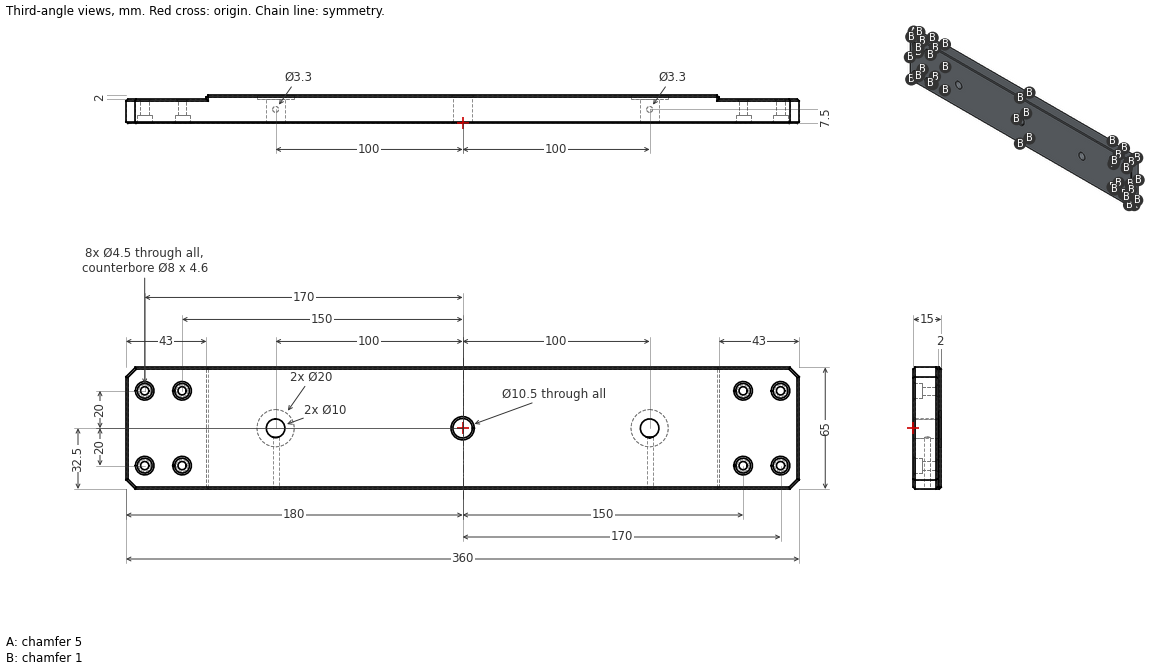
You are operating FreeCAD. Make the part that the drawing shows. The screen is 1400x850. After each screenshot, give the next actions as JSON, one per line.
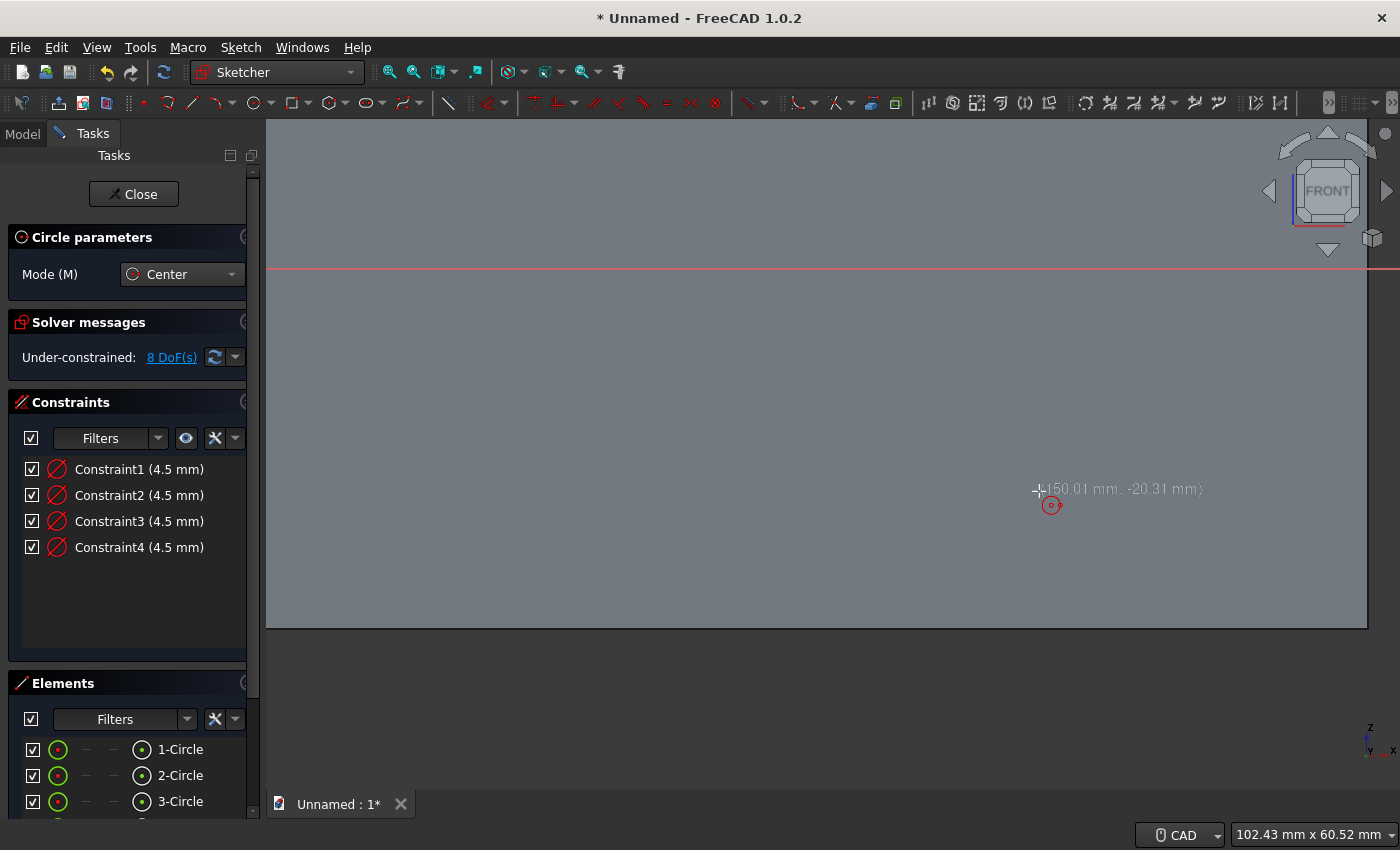
{"action": "scroll", "coordinate": [1040, 491], "scroll_direction": "down", "scroll_amount": 9}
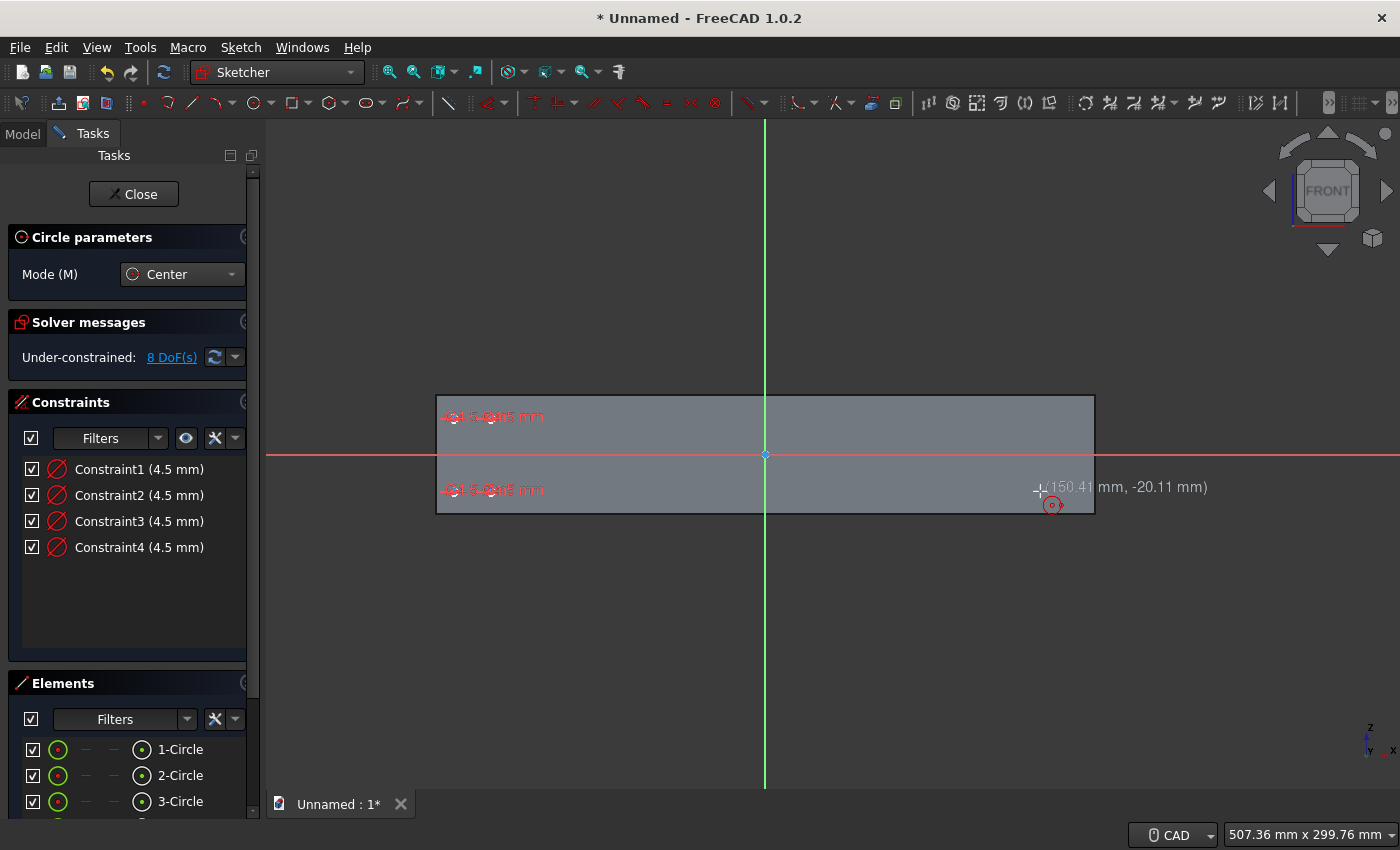
{"action": "left_click", "coordinate": [1040, 491]}
{"action": "mouse_move", "coordinate": [1043, 489]}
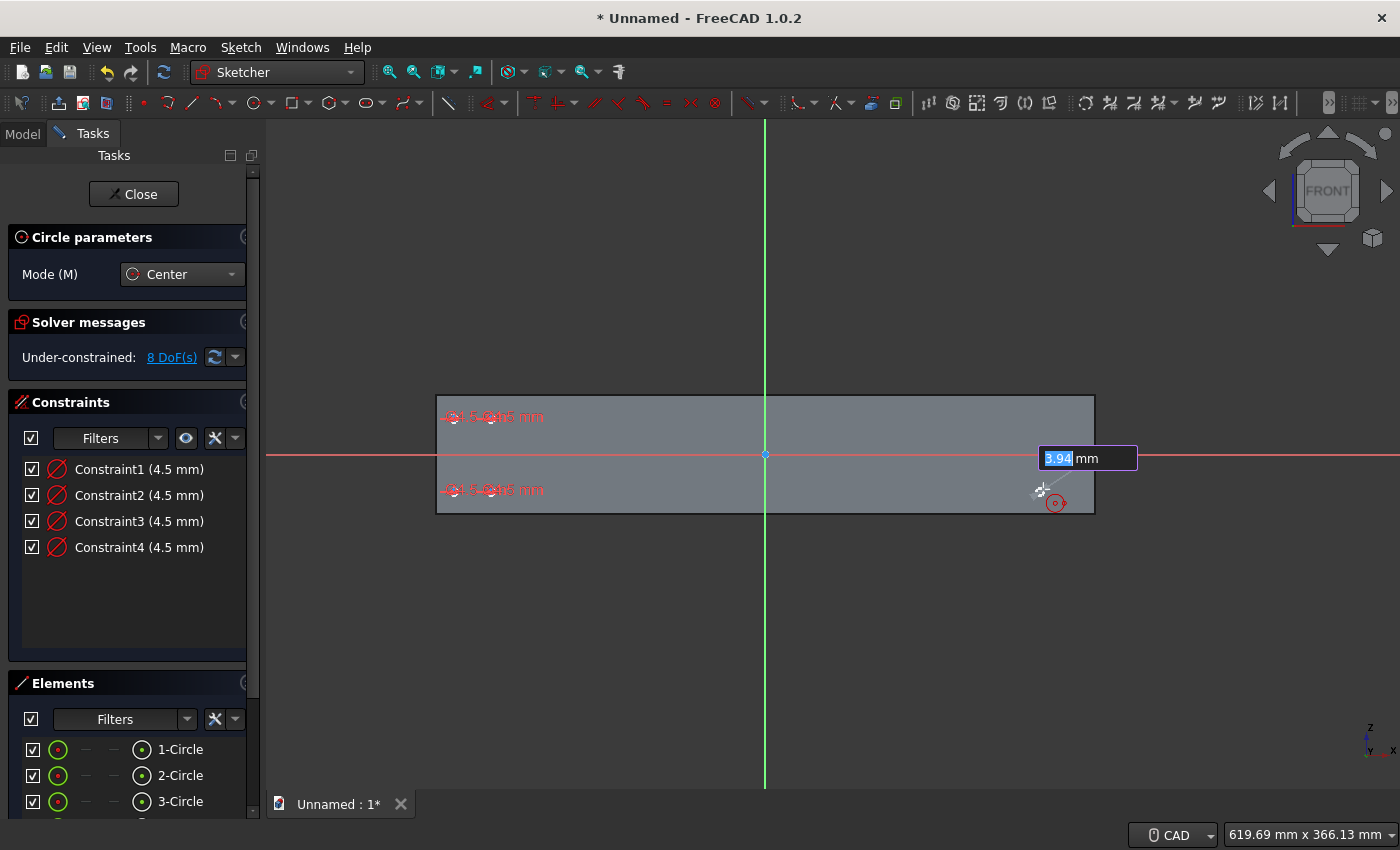
{"action": "type", "text": "4.5"}
{"action": "key", "text": "Return"}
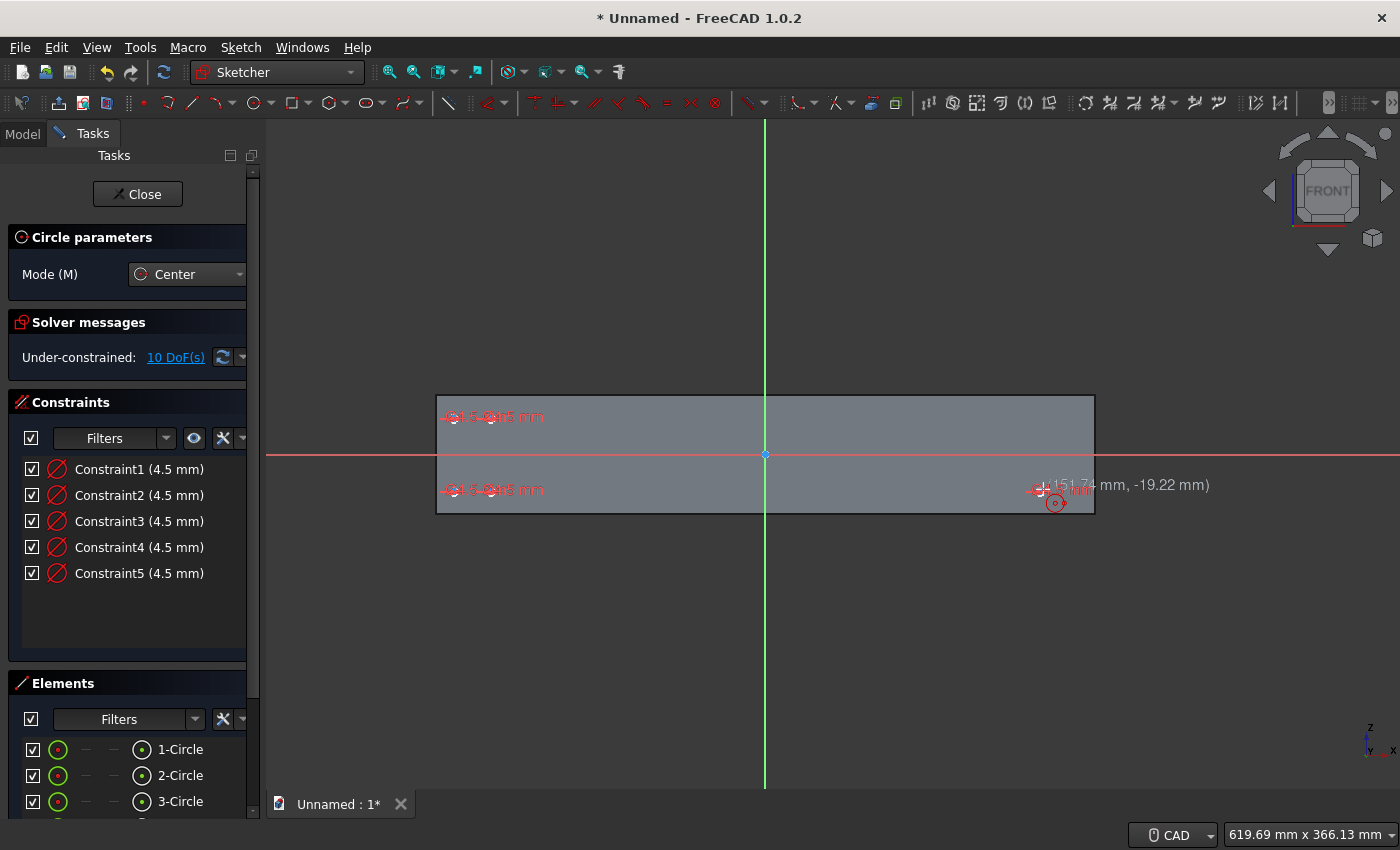
{"action": "scroll", "coordinate": [1076, 491], "scroll_direction": "up", "scroll_amount": 9}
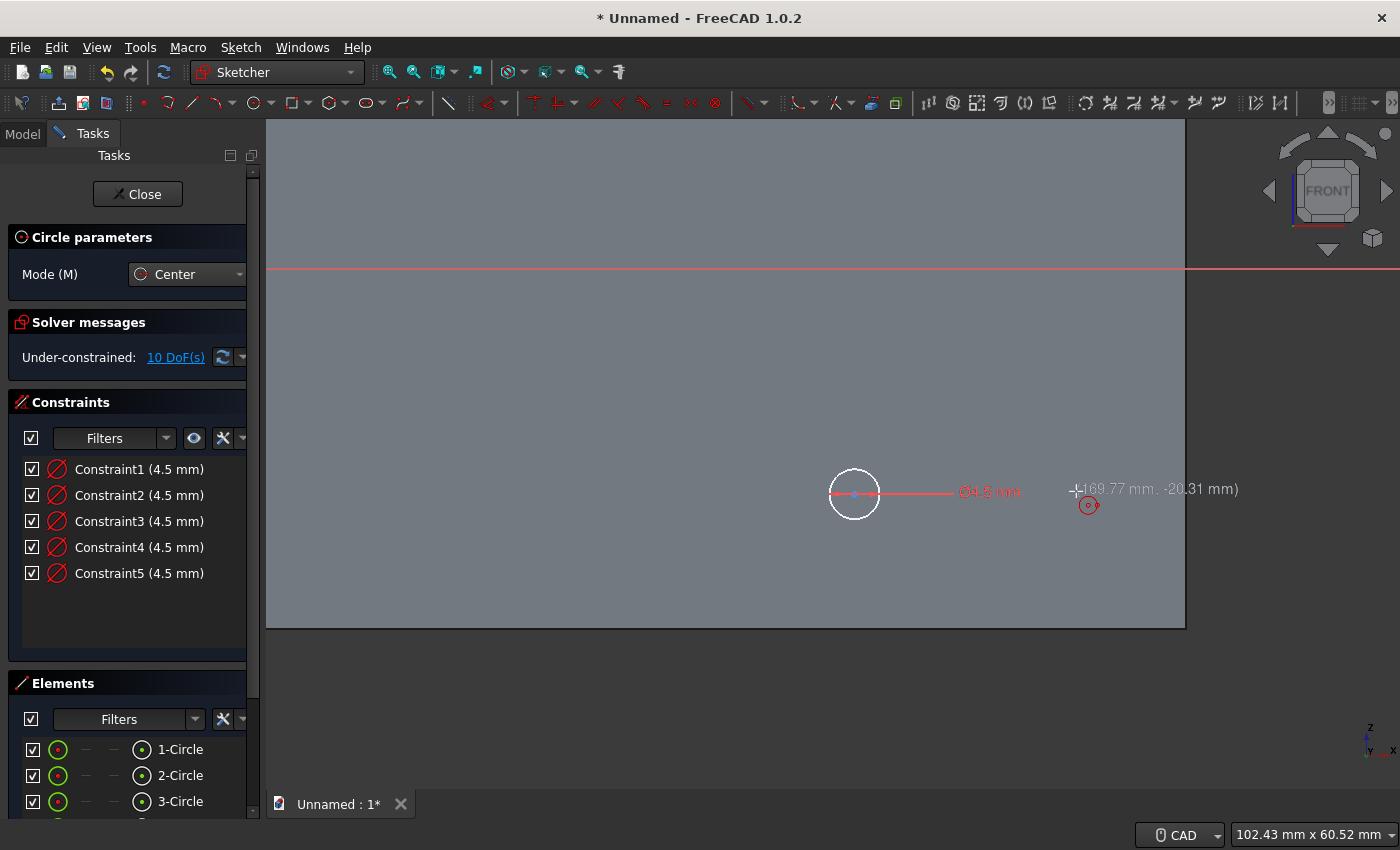
{"action": "scroll", "coordinate": [1076, 491], "scroll_direction": "down", "scroll_amount": 9}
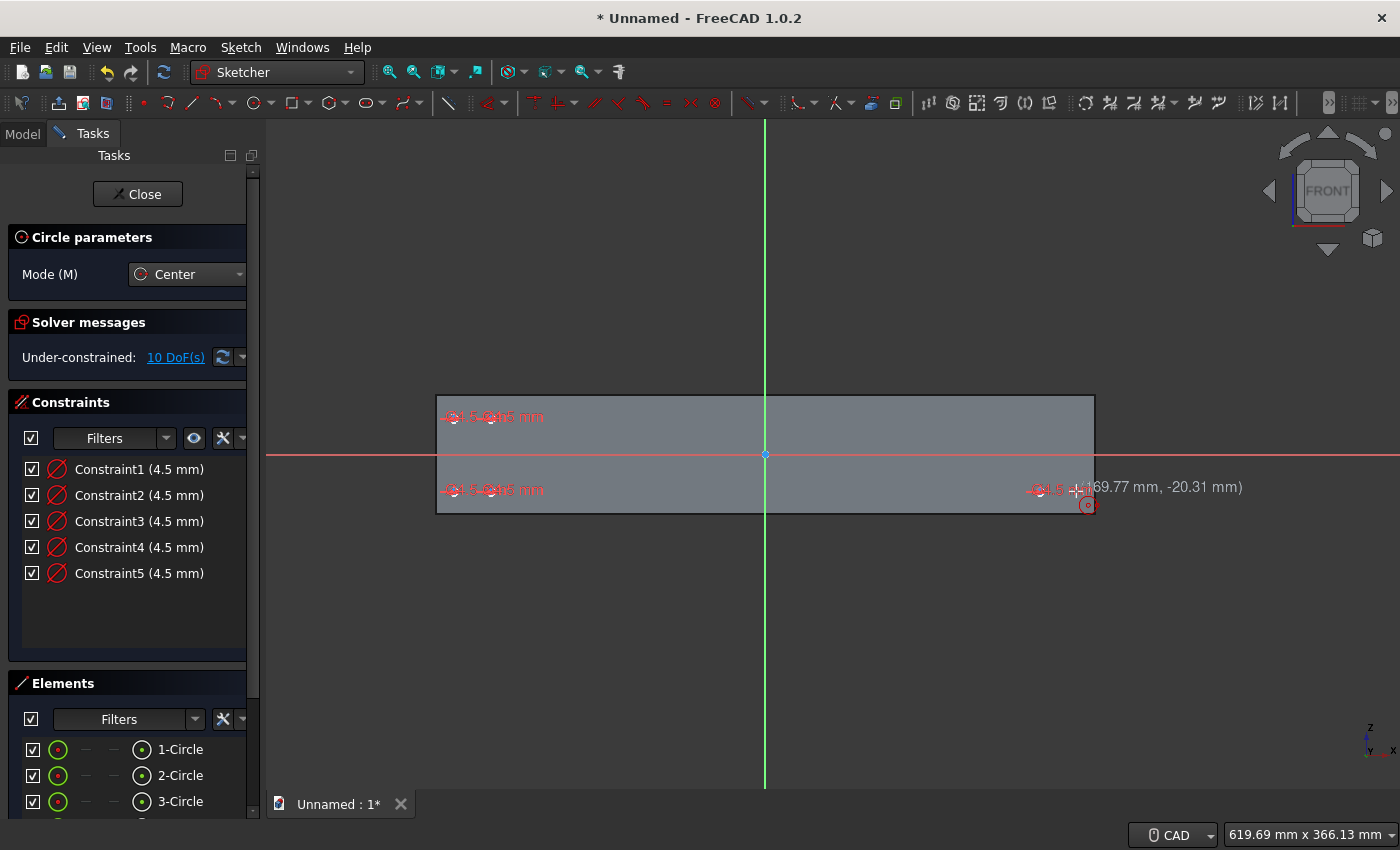
{"action": "left_click", "coordinate": [1076, 491]}
{"action": "mouse_move", "coordinate": [1079, 489]}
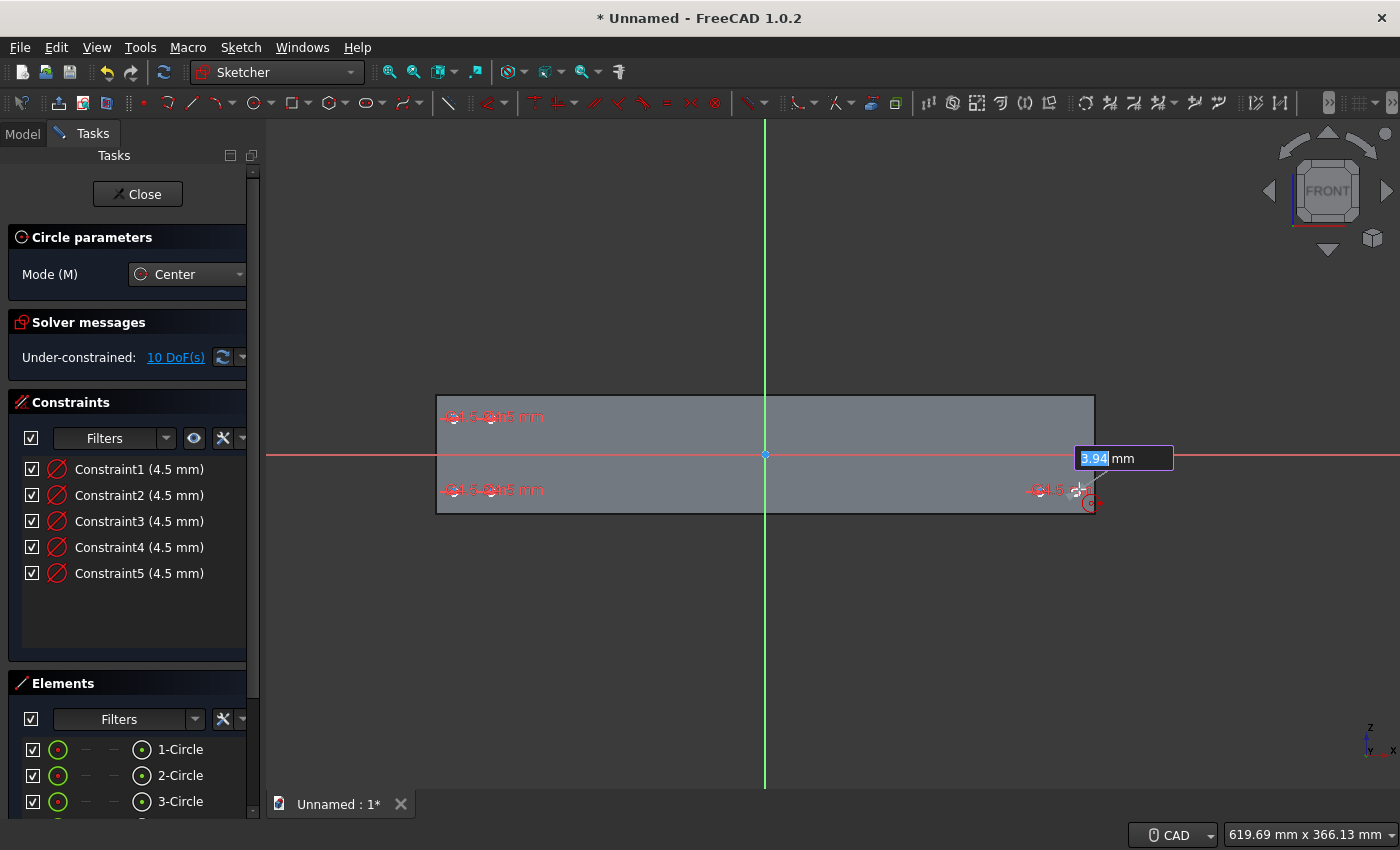
{"action": "type", "text": "4.5"}
{"action": "key", "text": "Return"}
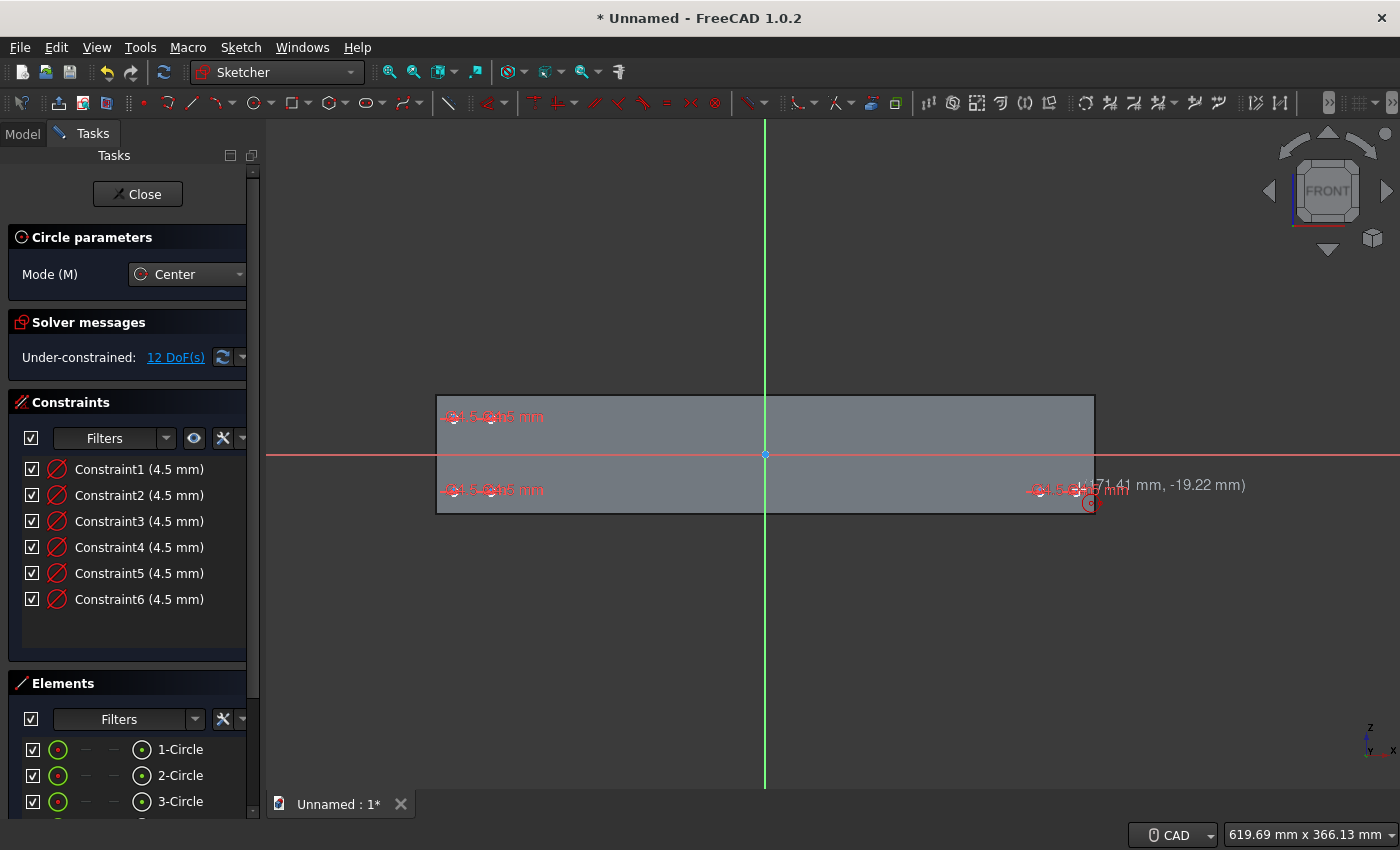
{"action": "scroll", "coordinate": [1040, 418], "scroll_direction": "up", "scroll_amount": 9}